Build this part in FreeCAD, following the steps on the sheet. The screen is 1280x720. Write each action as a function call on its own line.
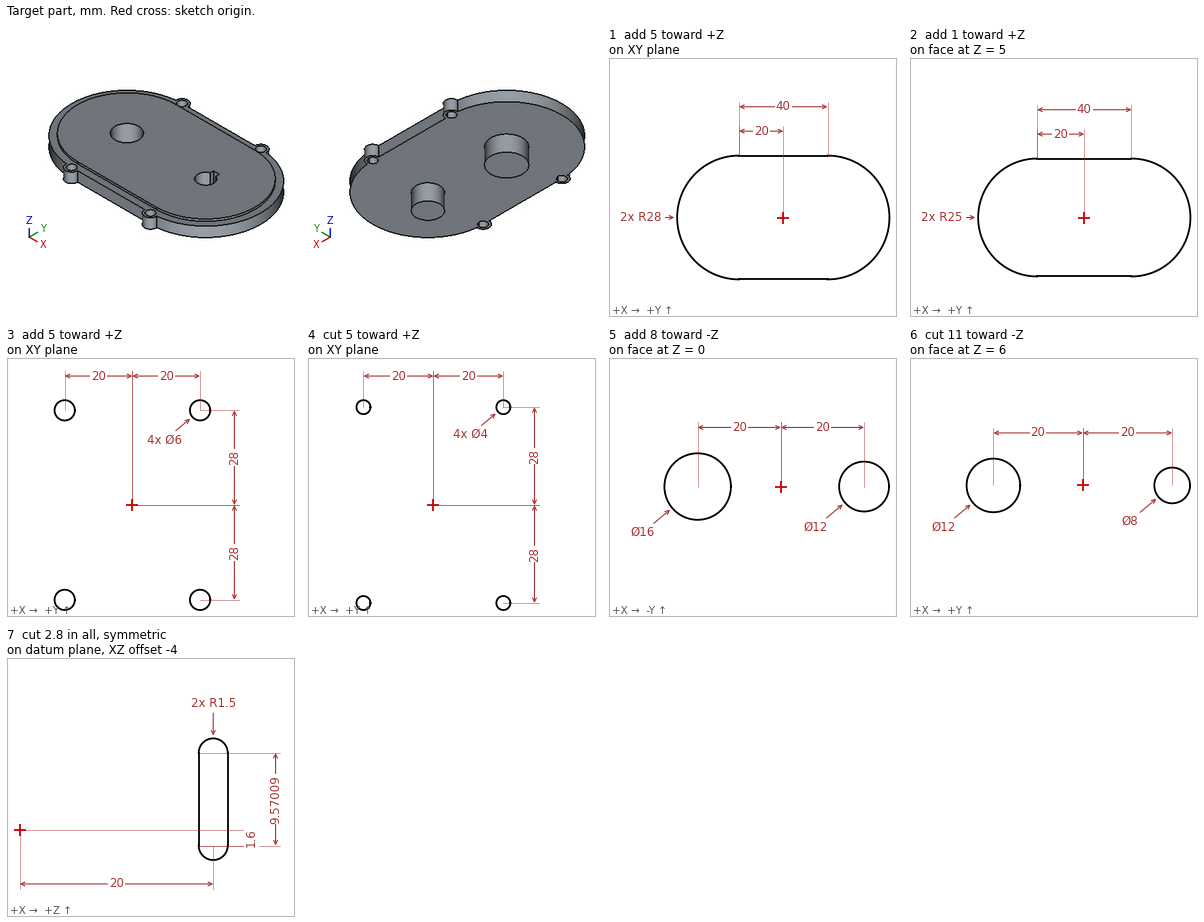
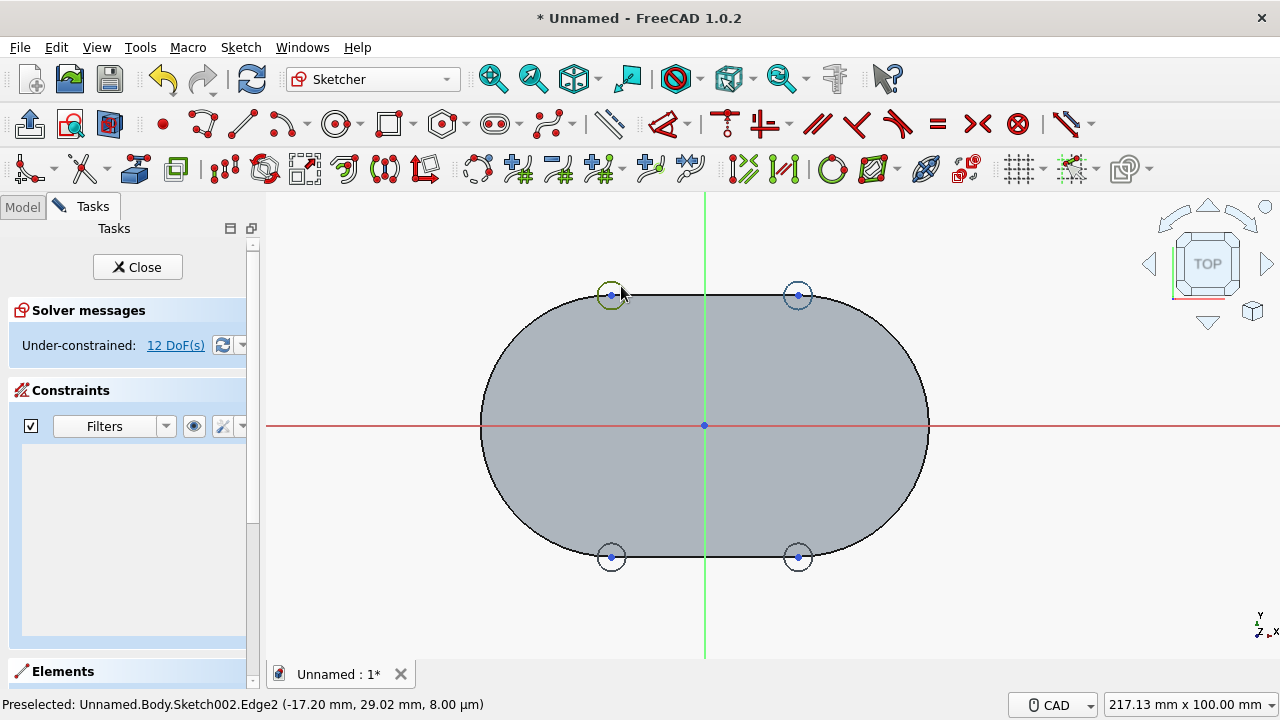
click(808, 547)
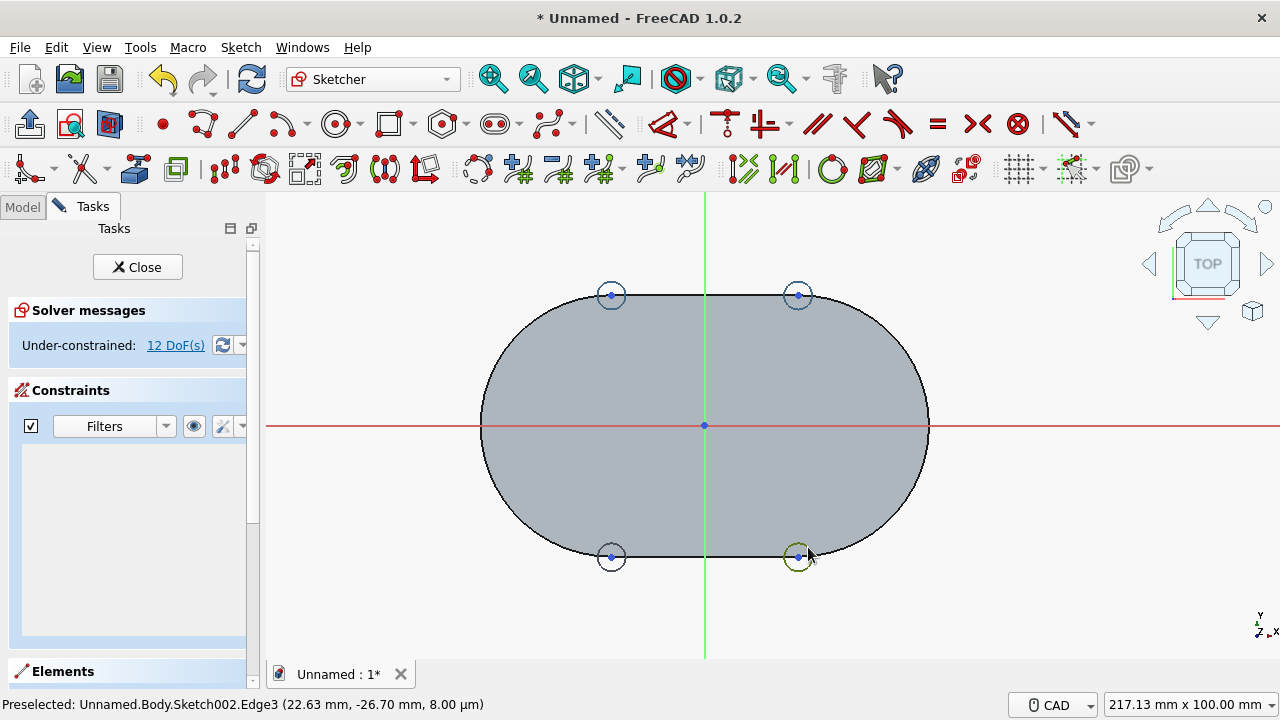
click(621, 547)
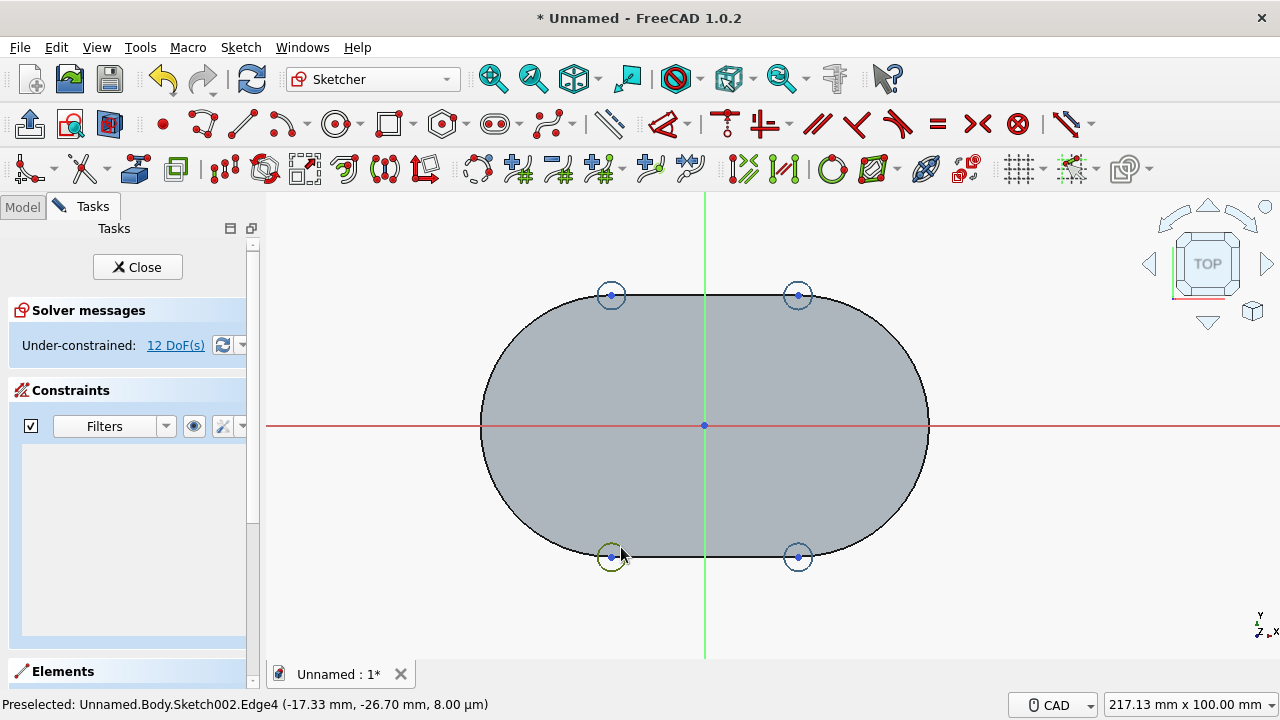
click(938, 124)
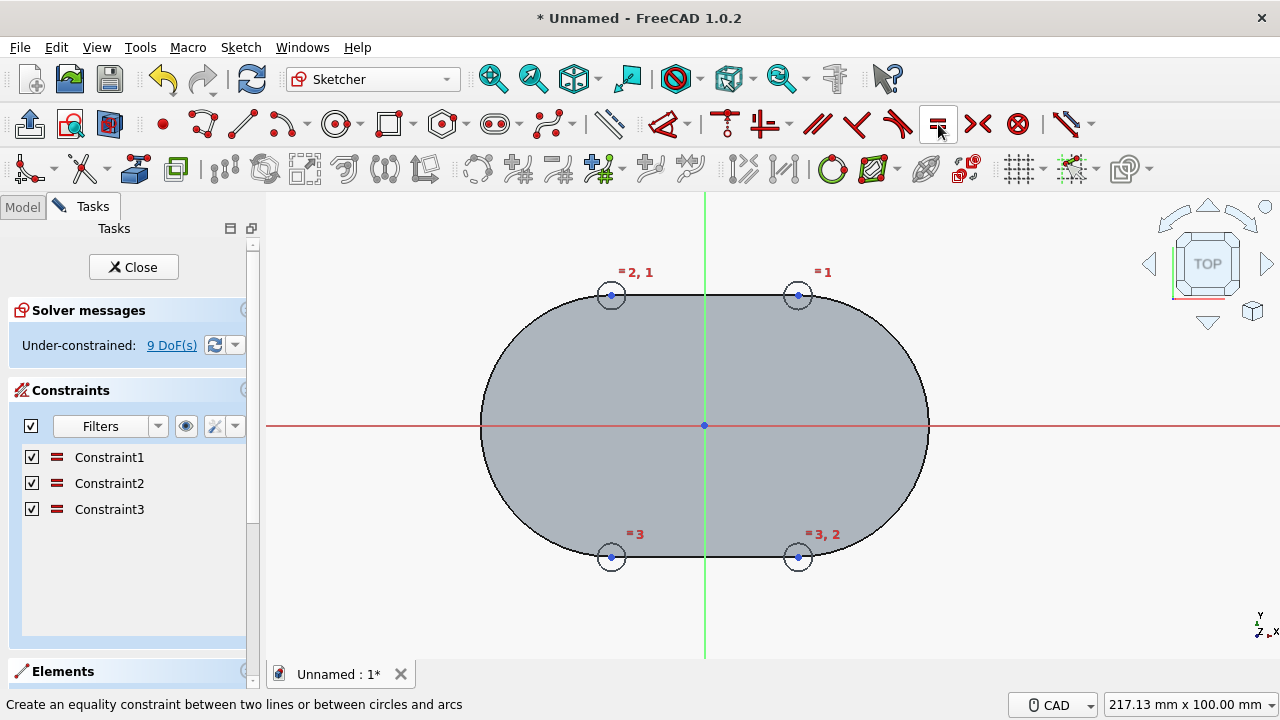
click(798, 296)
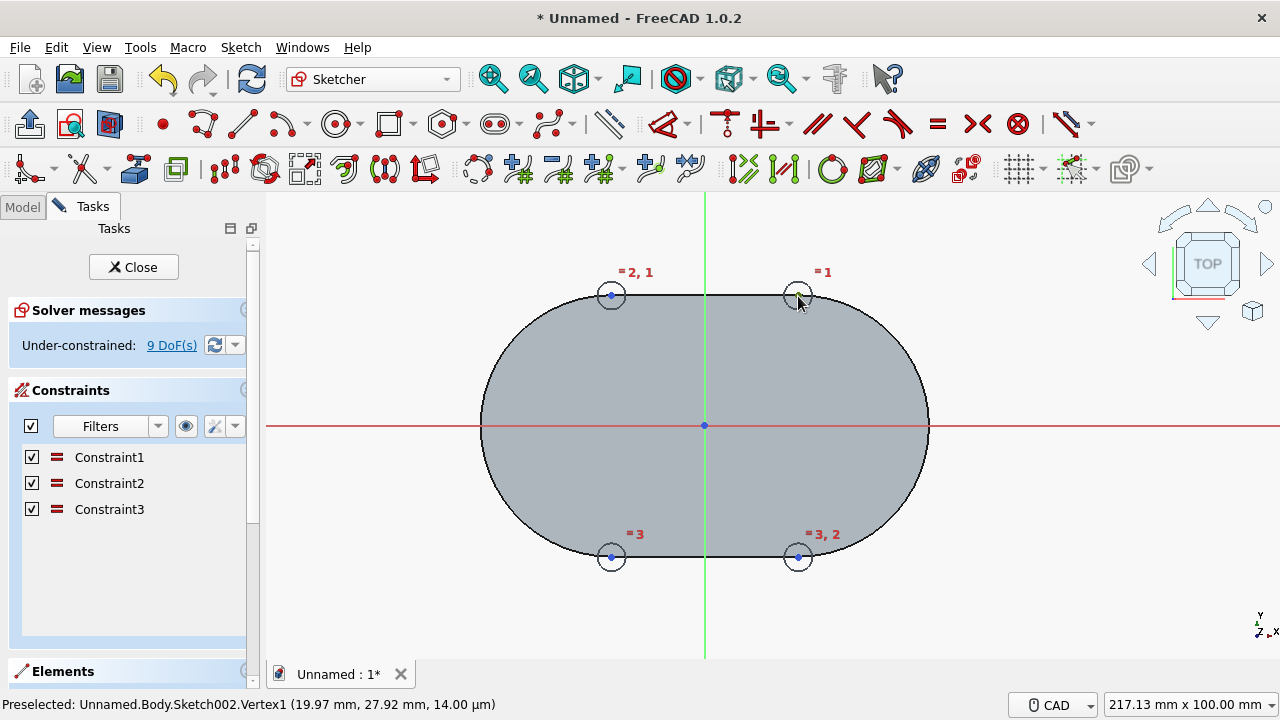
click(611, 296)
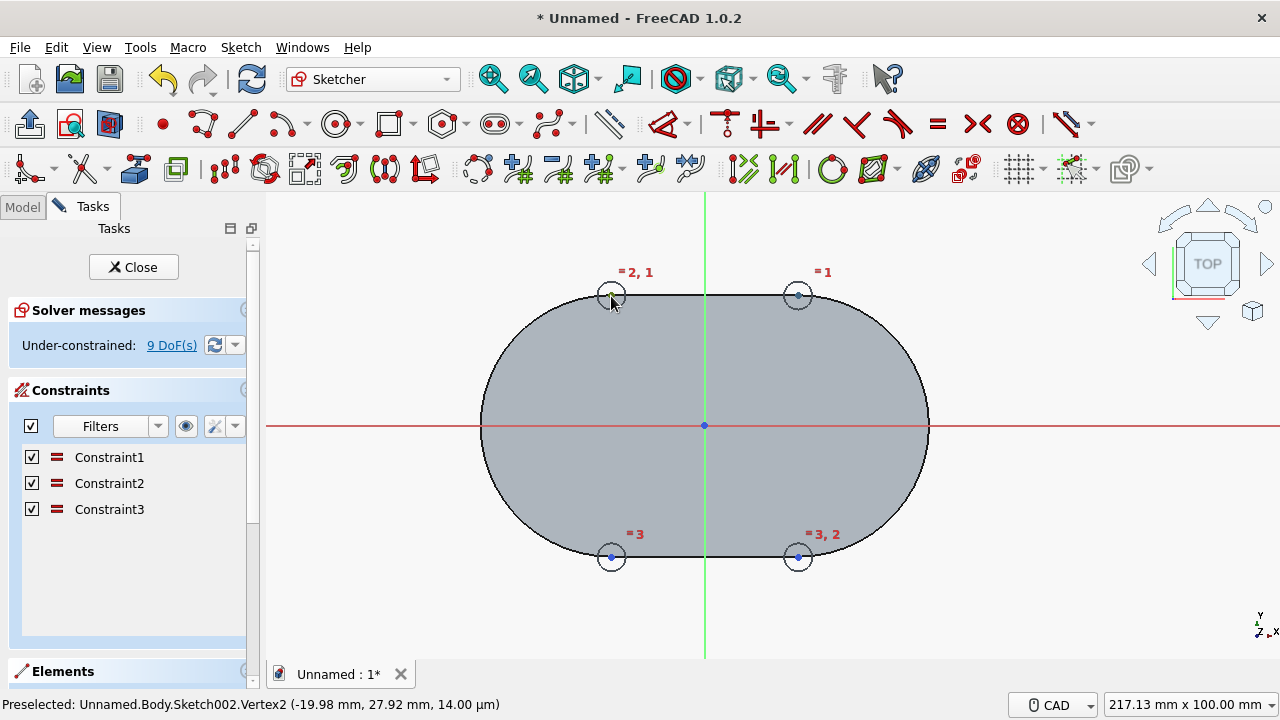
key(h)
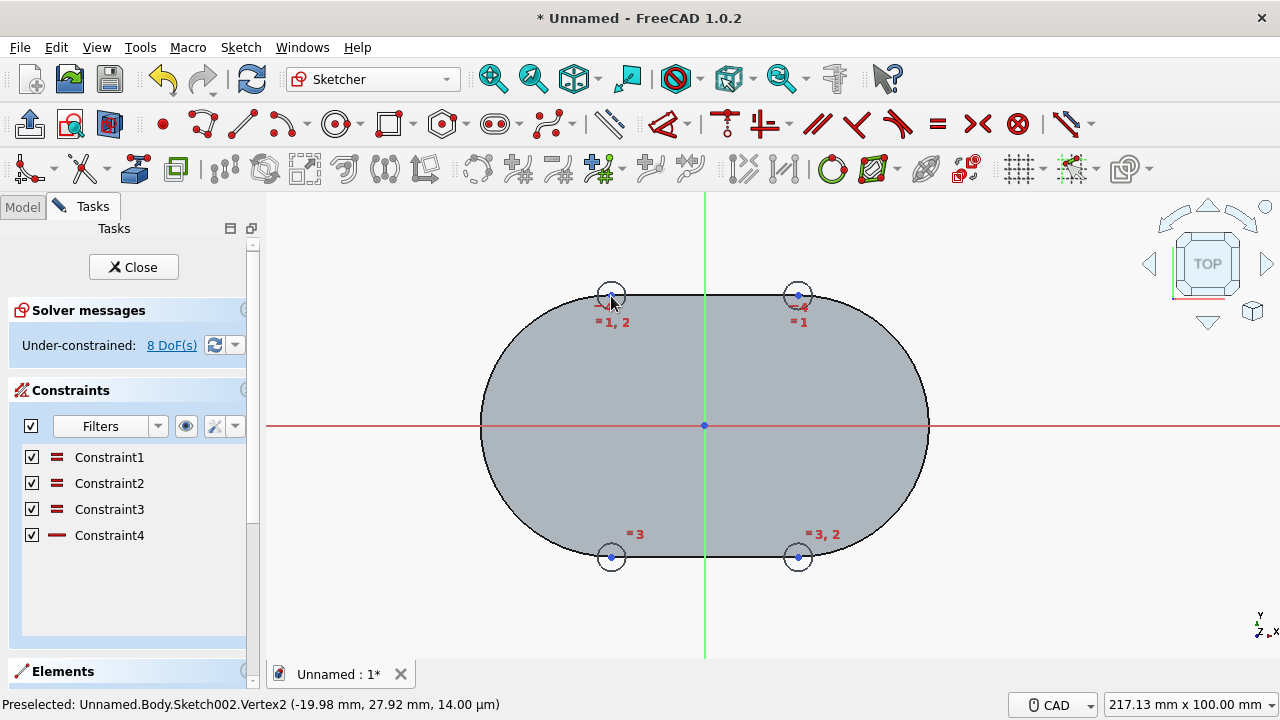
click(798, 296)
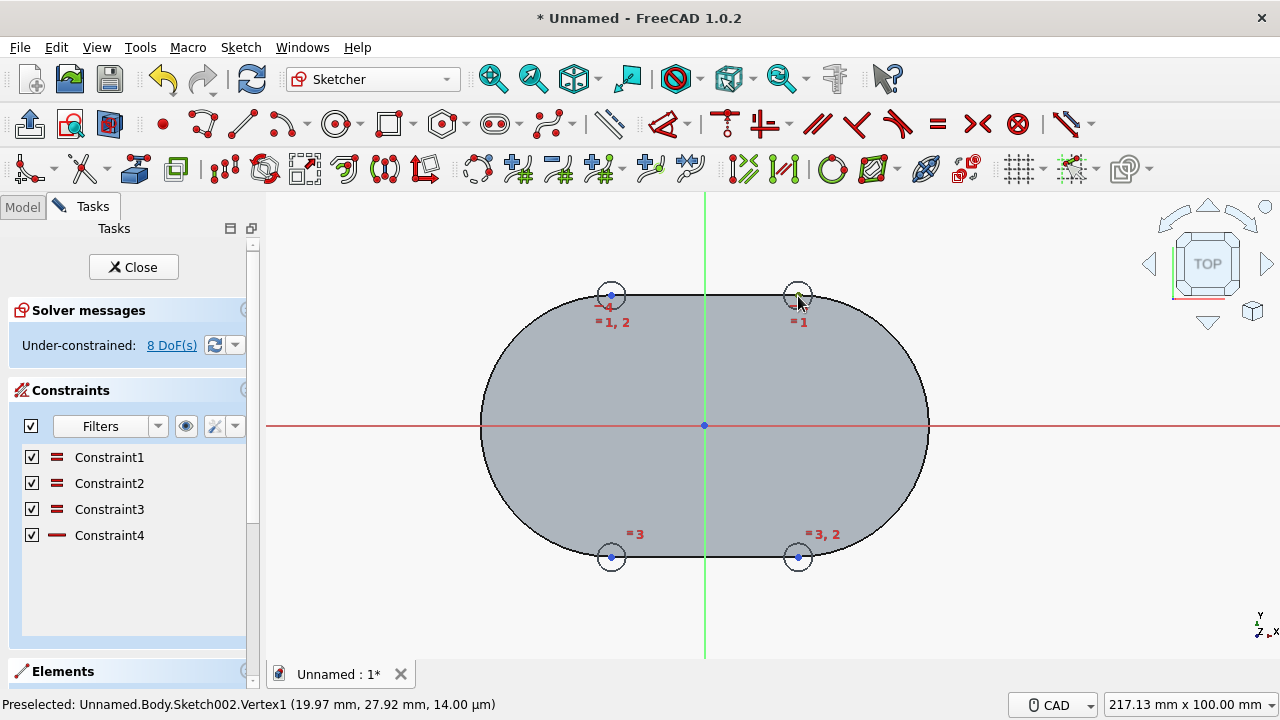
click(798, 557)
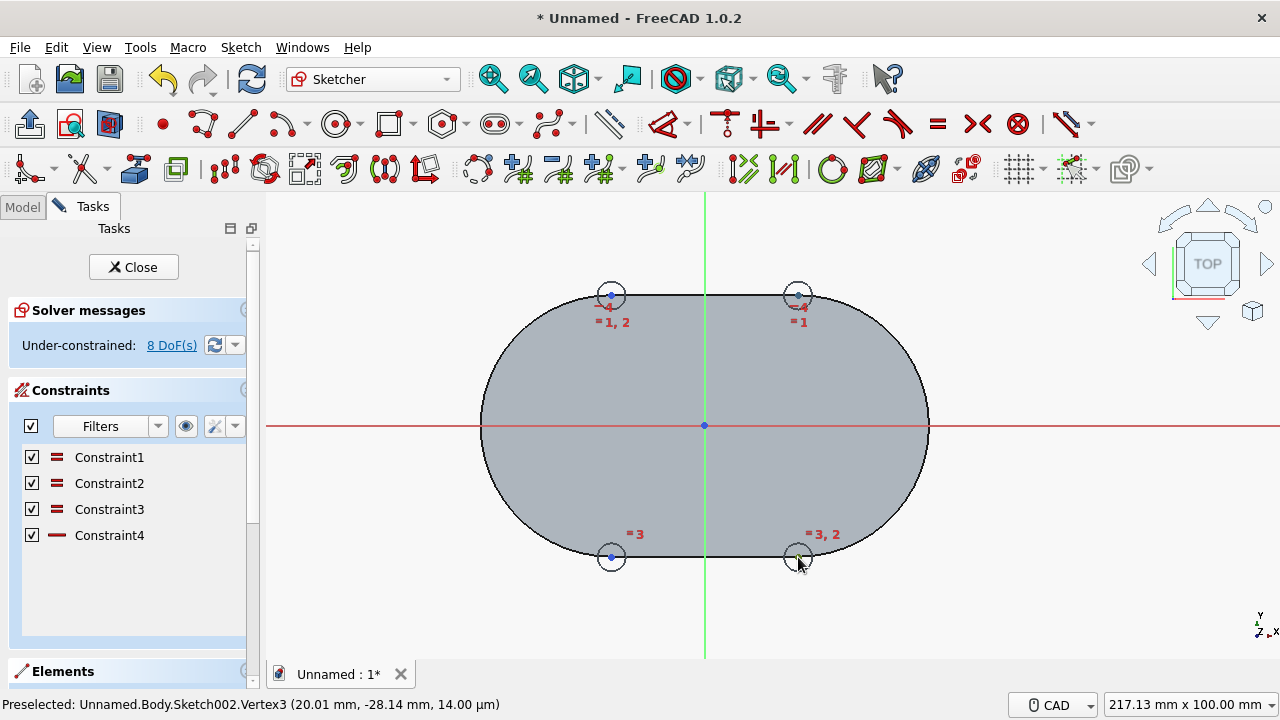
key(v)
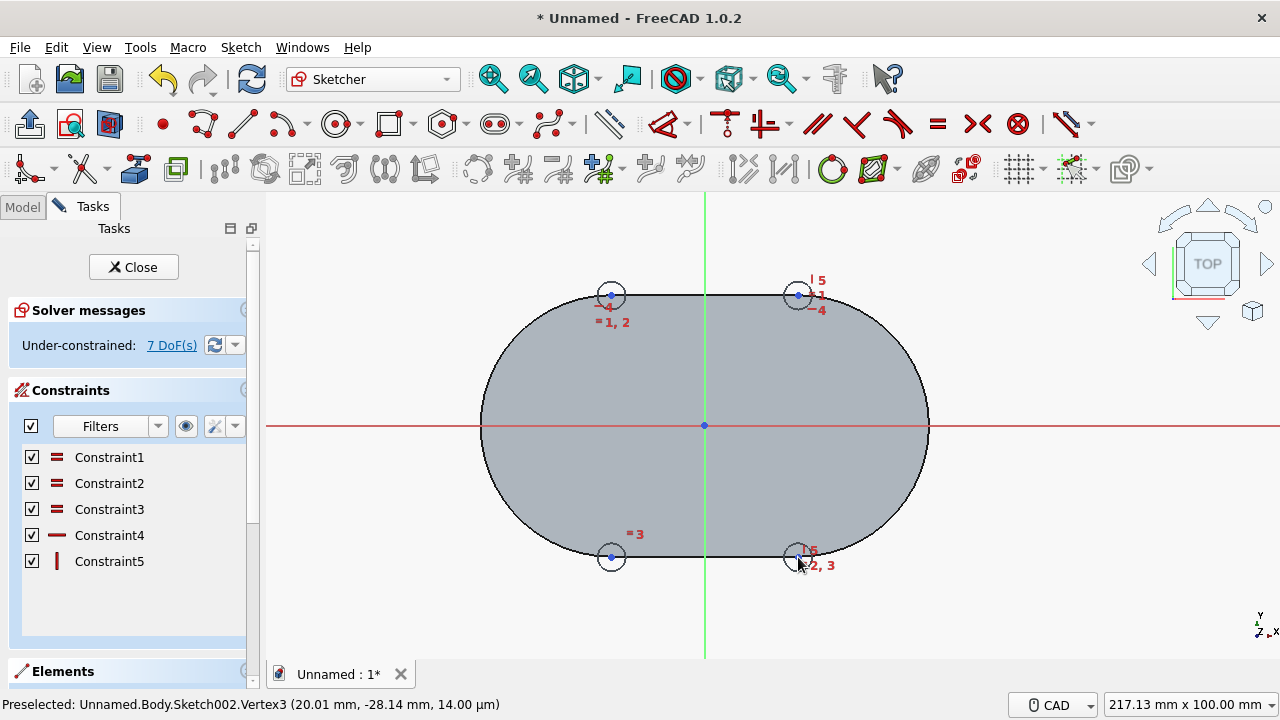
click(611, 296)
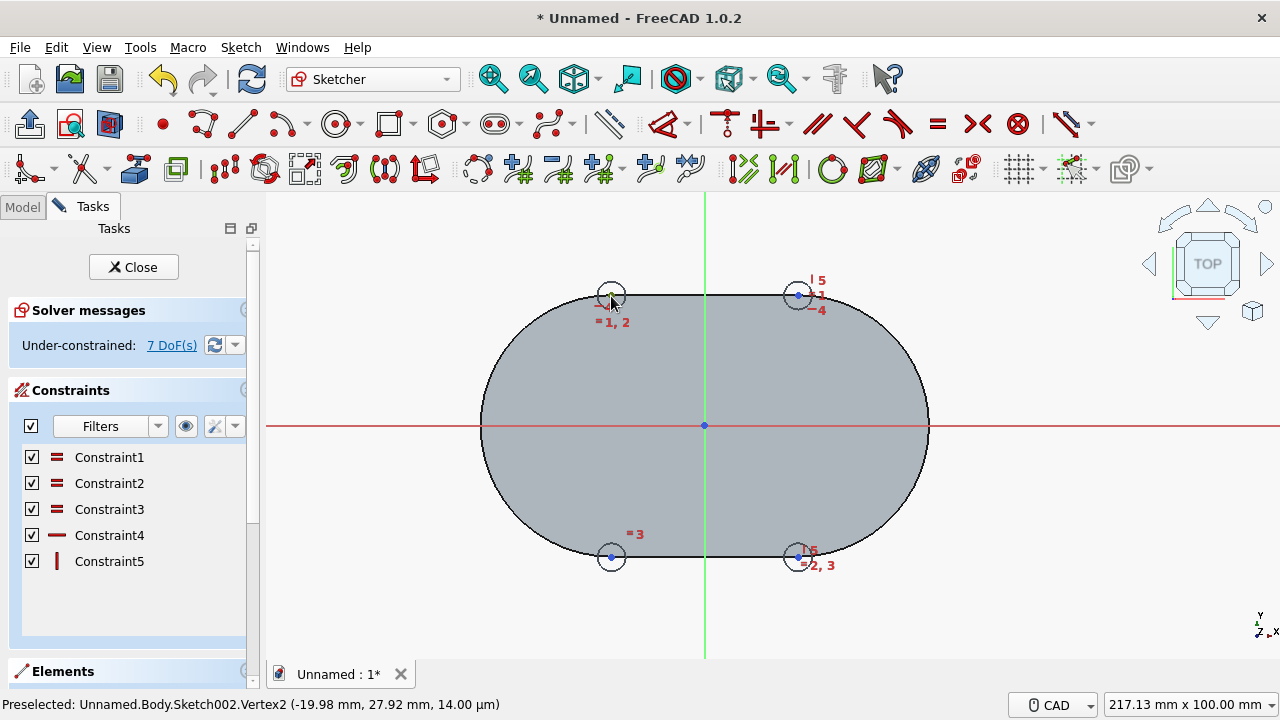
click(612, 557)